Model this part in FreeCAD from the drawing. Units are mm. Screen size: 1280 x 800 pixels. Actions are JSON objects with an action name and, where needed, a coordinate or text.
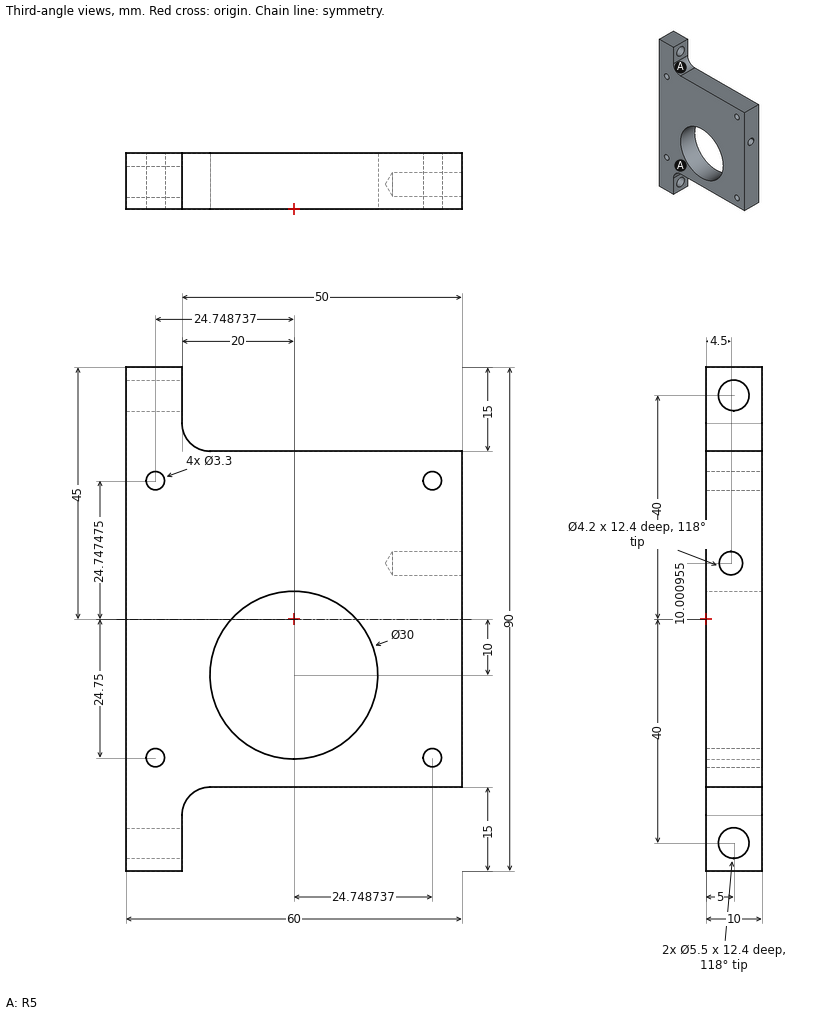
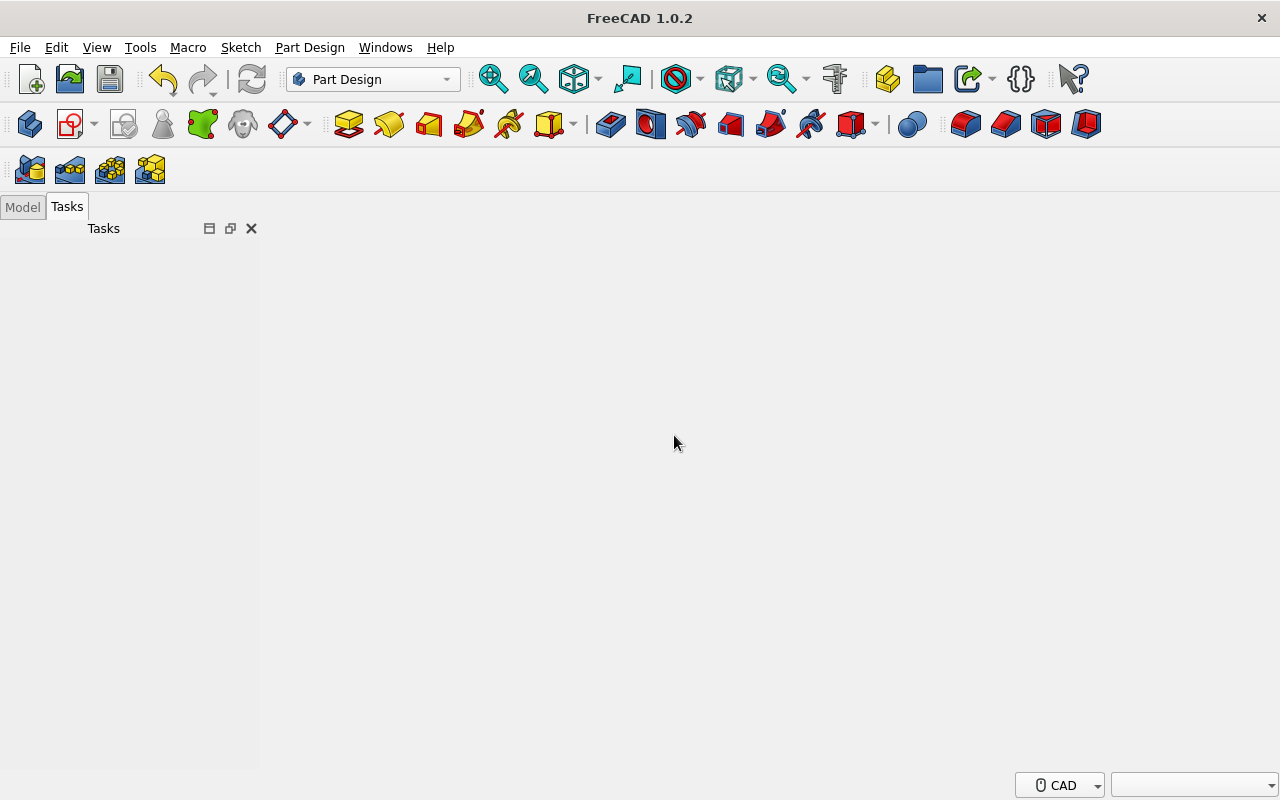
{"action": "left_click", "coordinate": [30, 80]}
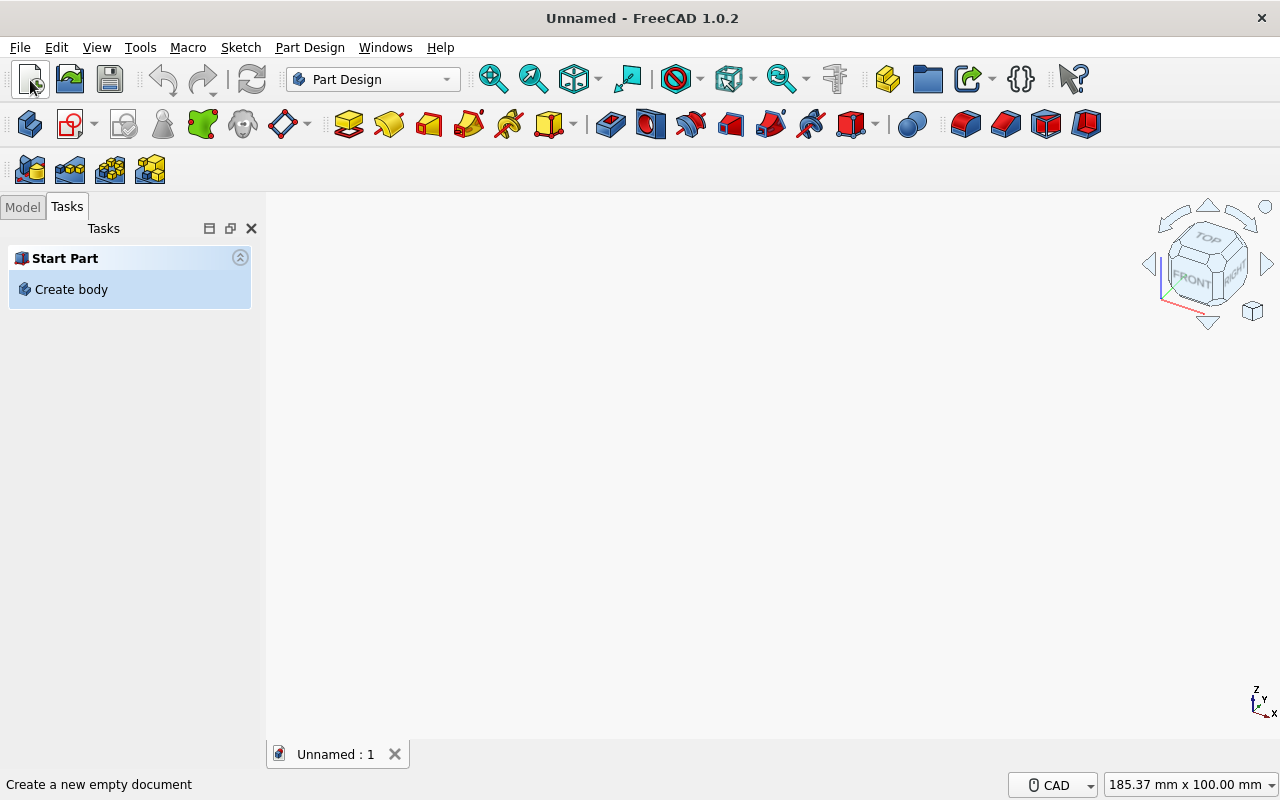
{"action": "left_click", "coordinate": [70, 124]}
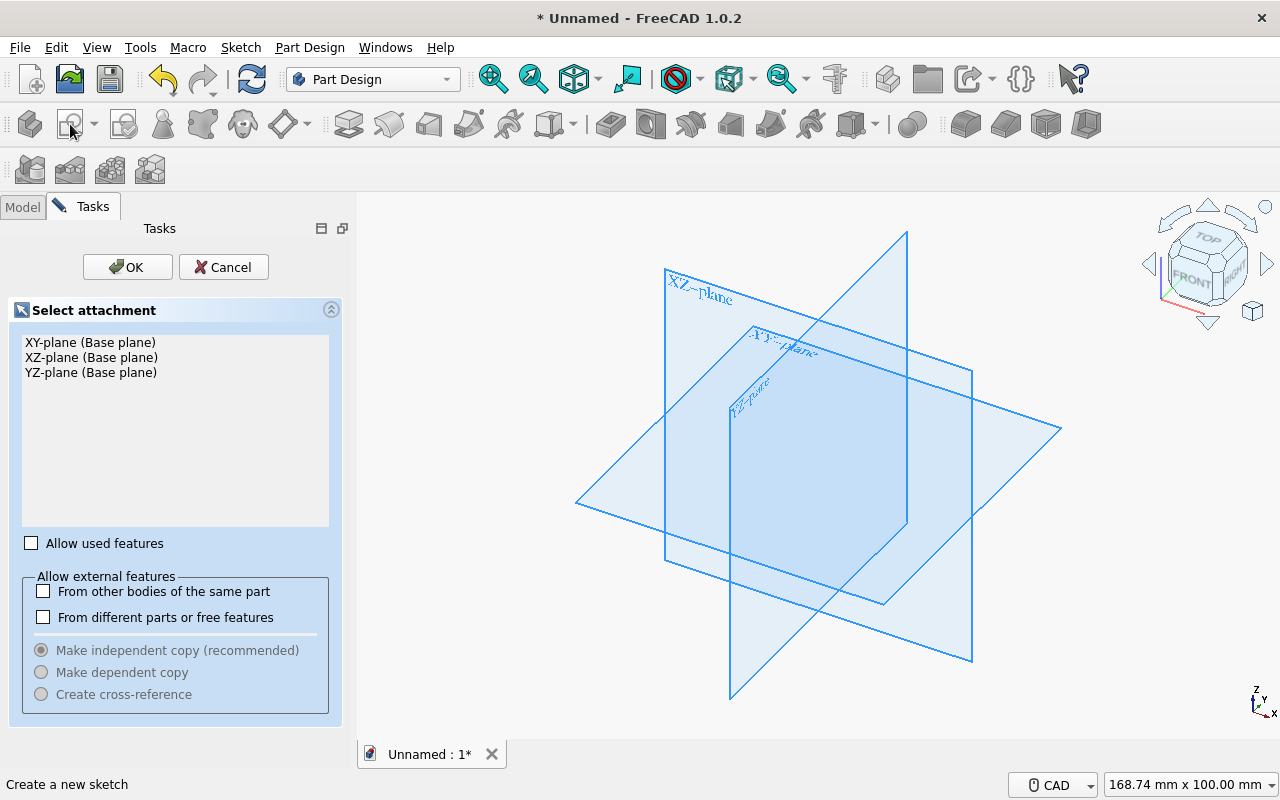
{"action": "left_click", "coordinate": [82, 358]}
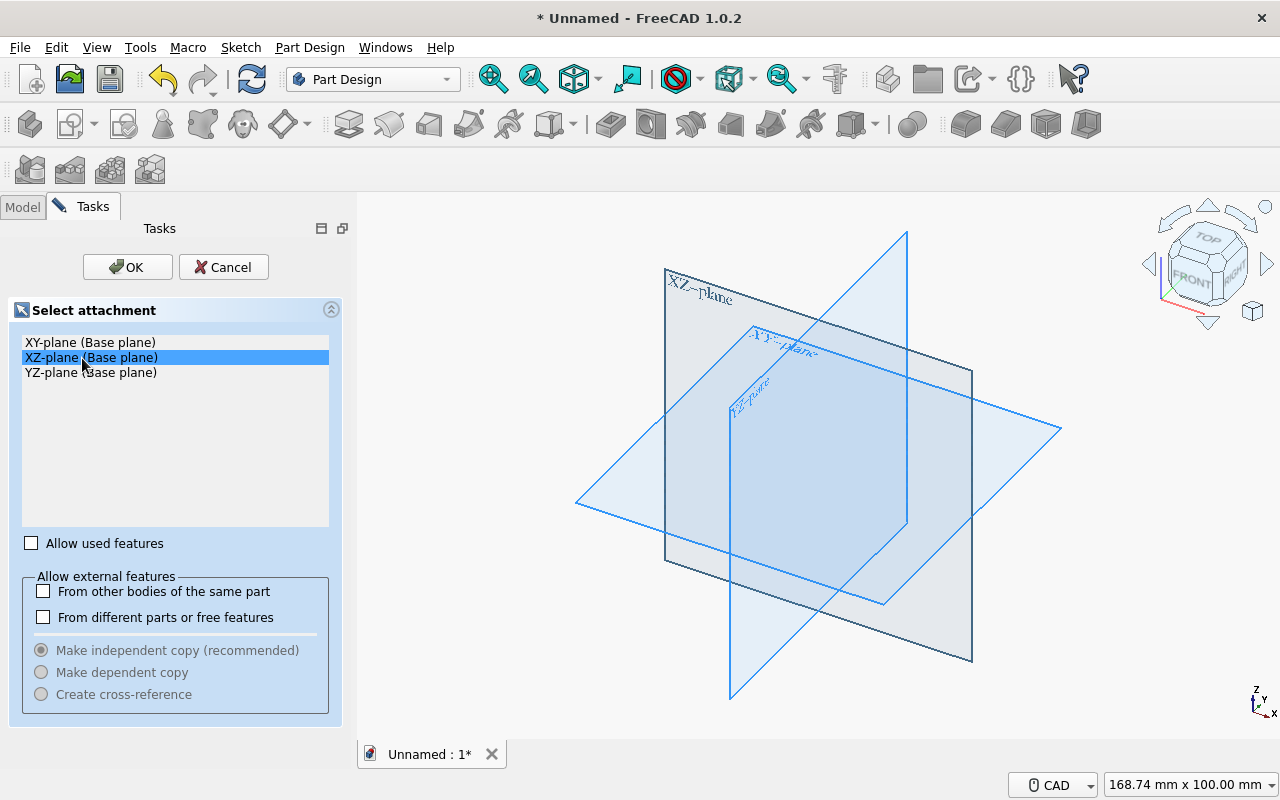
{"action": "left_click", "coordinate": [128, 267]}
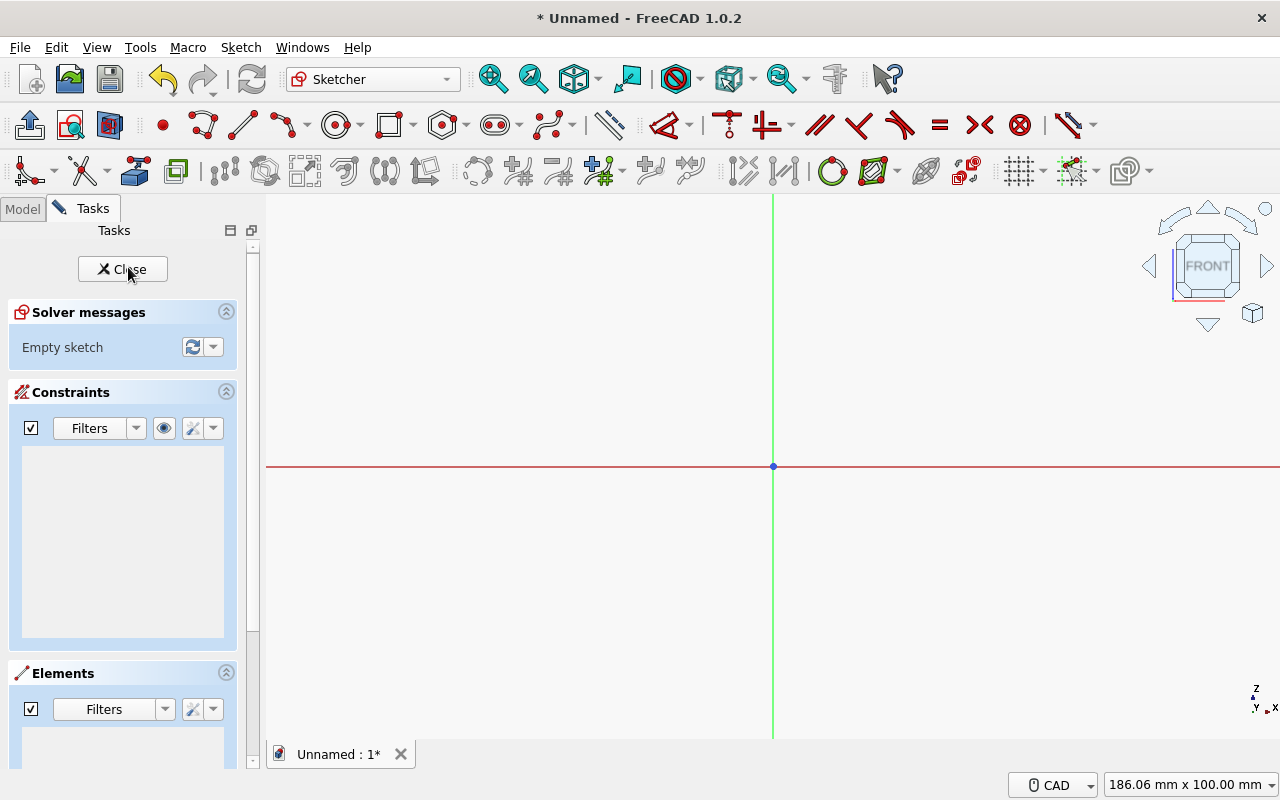
{"action": "scroll", "coordinate": [565, 466], "scroll_direction": "down", "scroll_amount": 2}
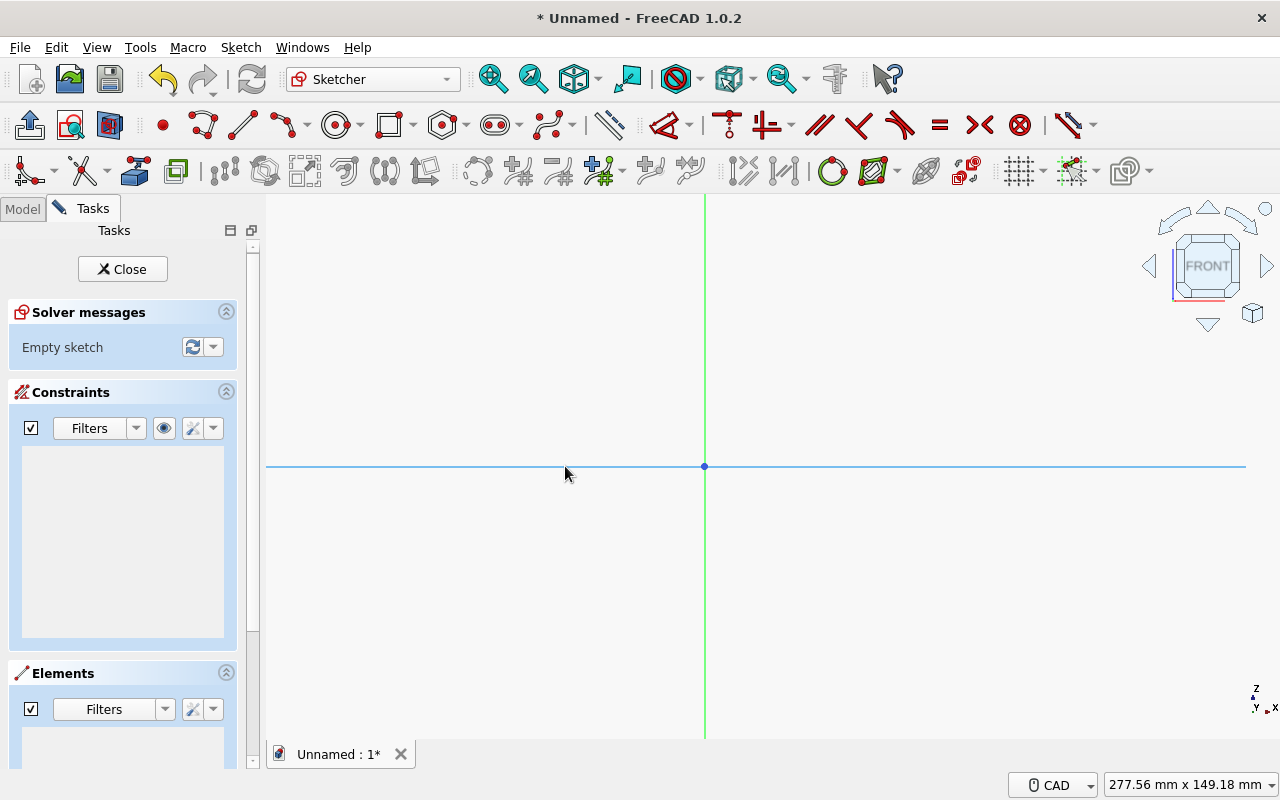
{"action": "key", "text": "g v"}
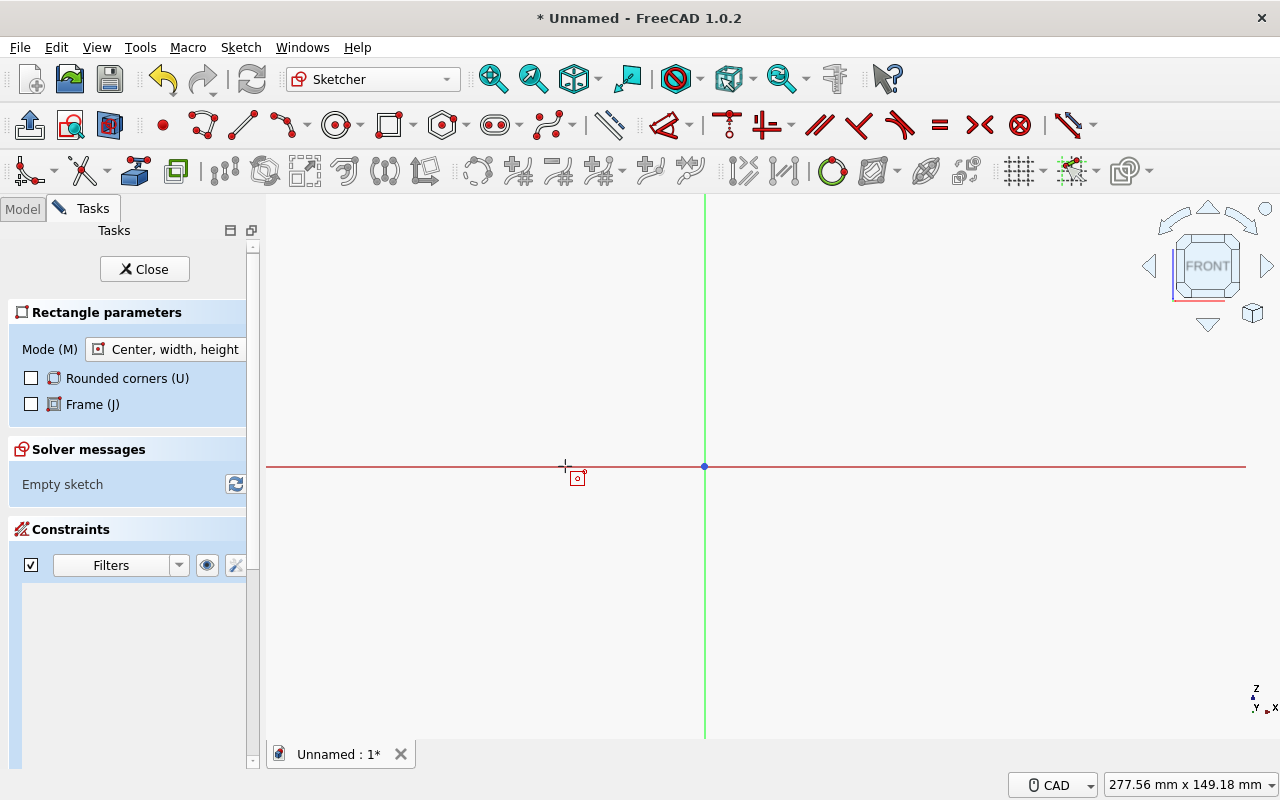
{"action": "left_click", "coordinate": [705, 466]}
{"action": "mouse_move", "coordinate": [814, 302]}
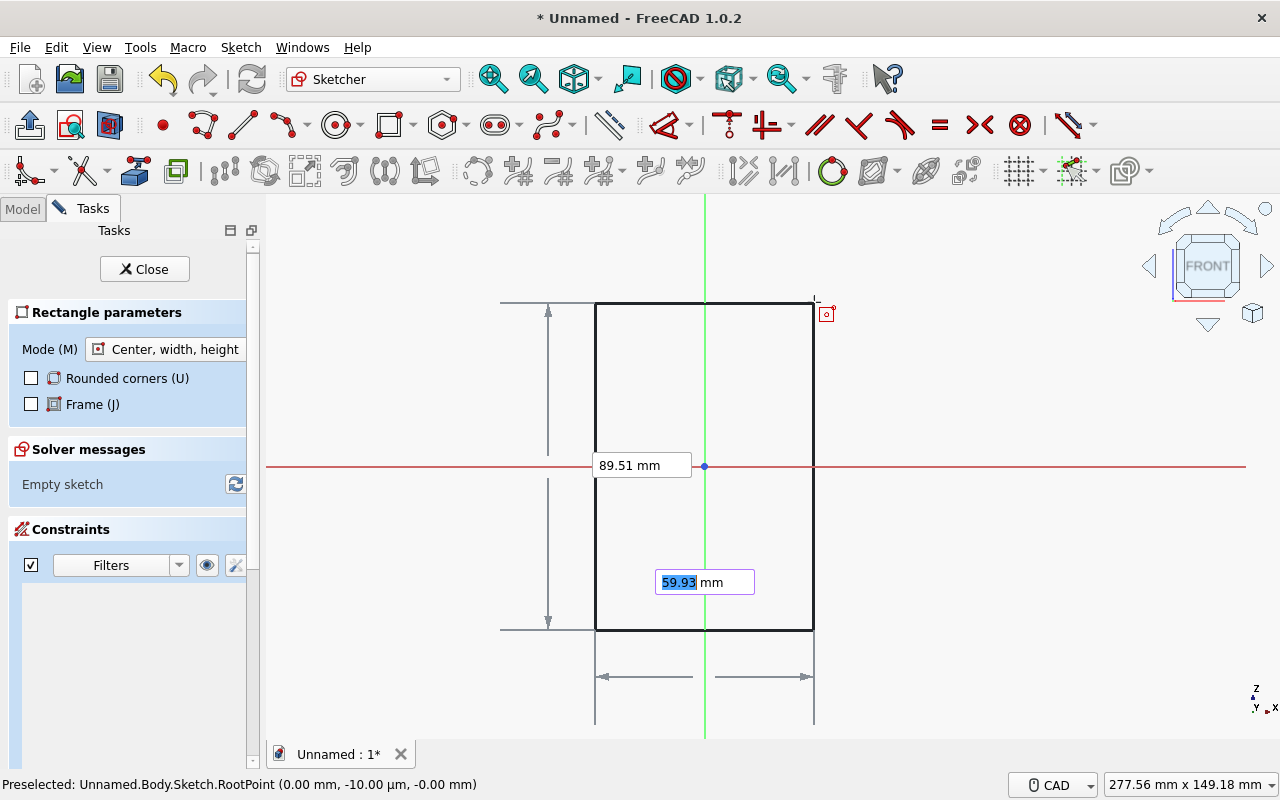
{"action": "type", "text": "60"}
{"action": "key", "text": "Tab"}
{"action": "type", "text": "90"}
{"action": "key", "text": "Return"}
{"action": "key", "text": "Escape"}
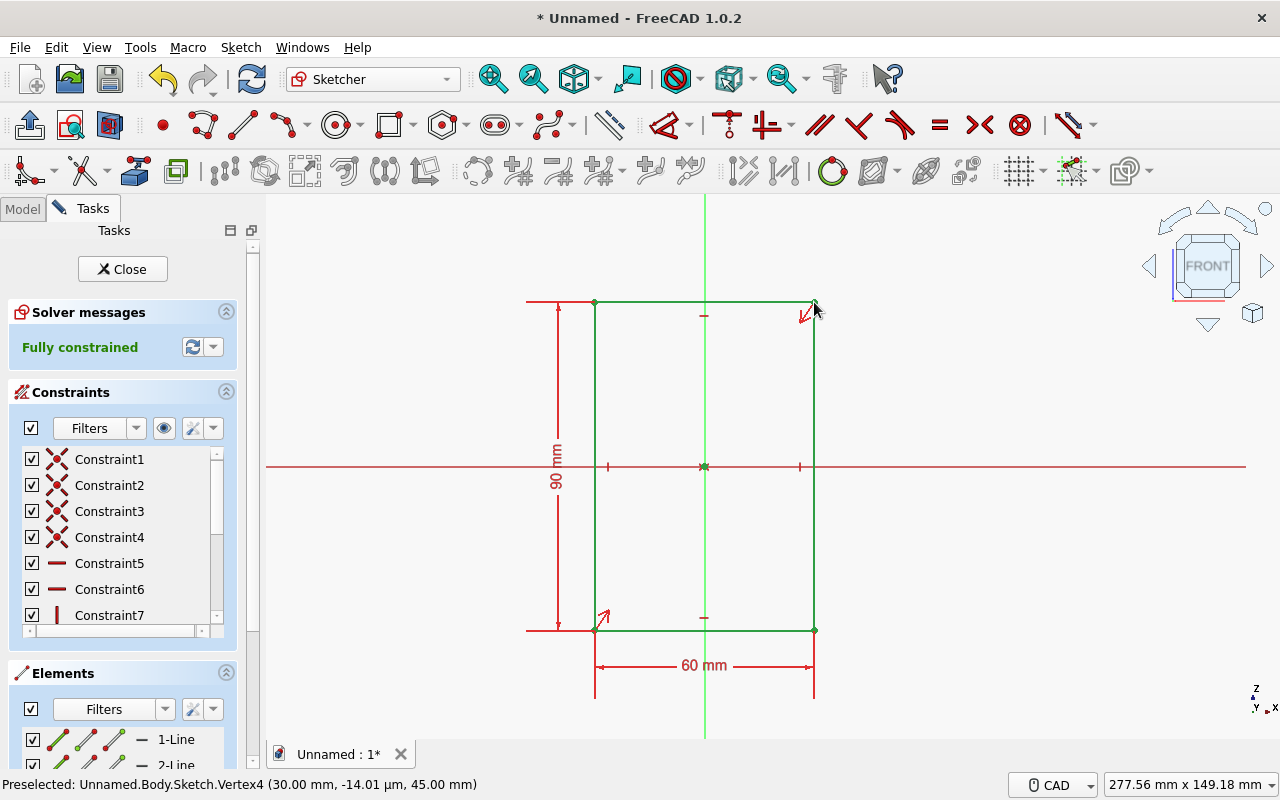
{"action": "left_click", "coordinate": [123, 269]}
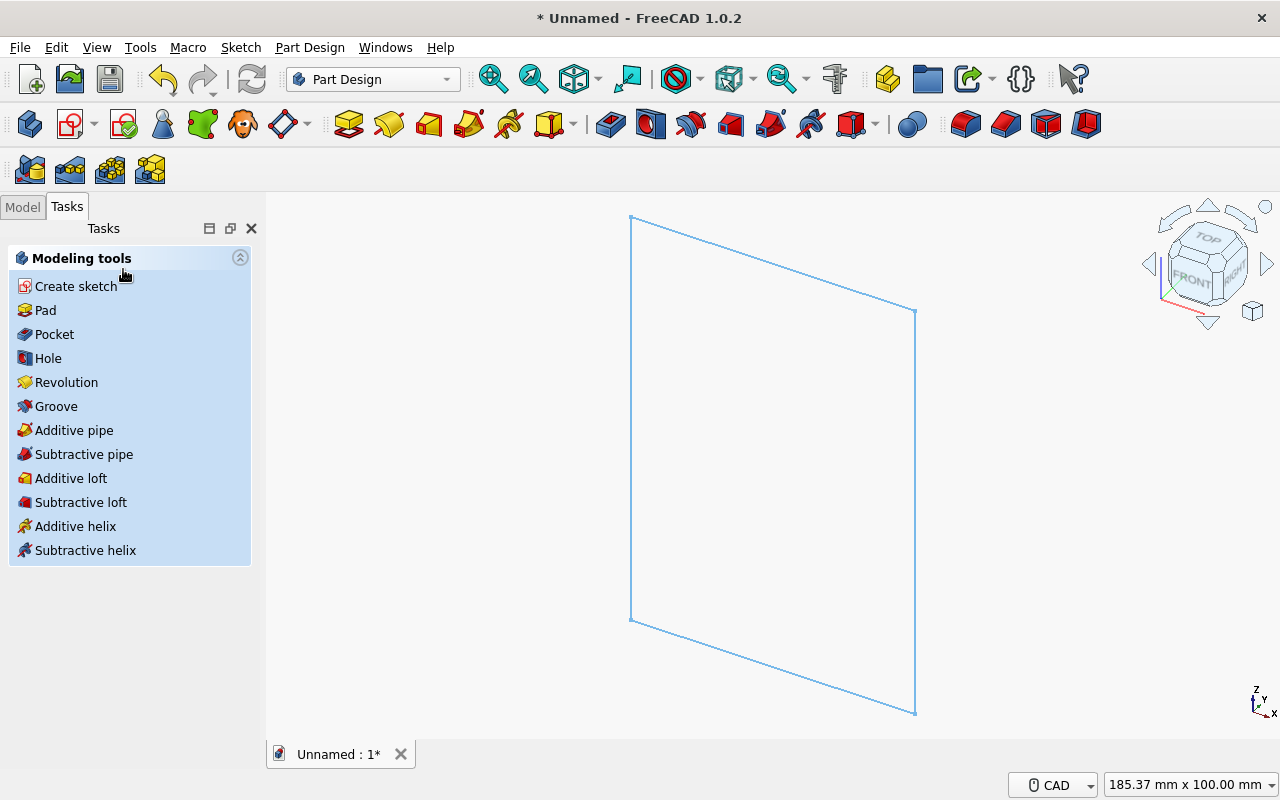
{"action": "left_click", "coordinate": [350, 124]}